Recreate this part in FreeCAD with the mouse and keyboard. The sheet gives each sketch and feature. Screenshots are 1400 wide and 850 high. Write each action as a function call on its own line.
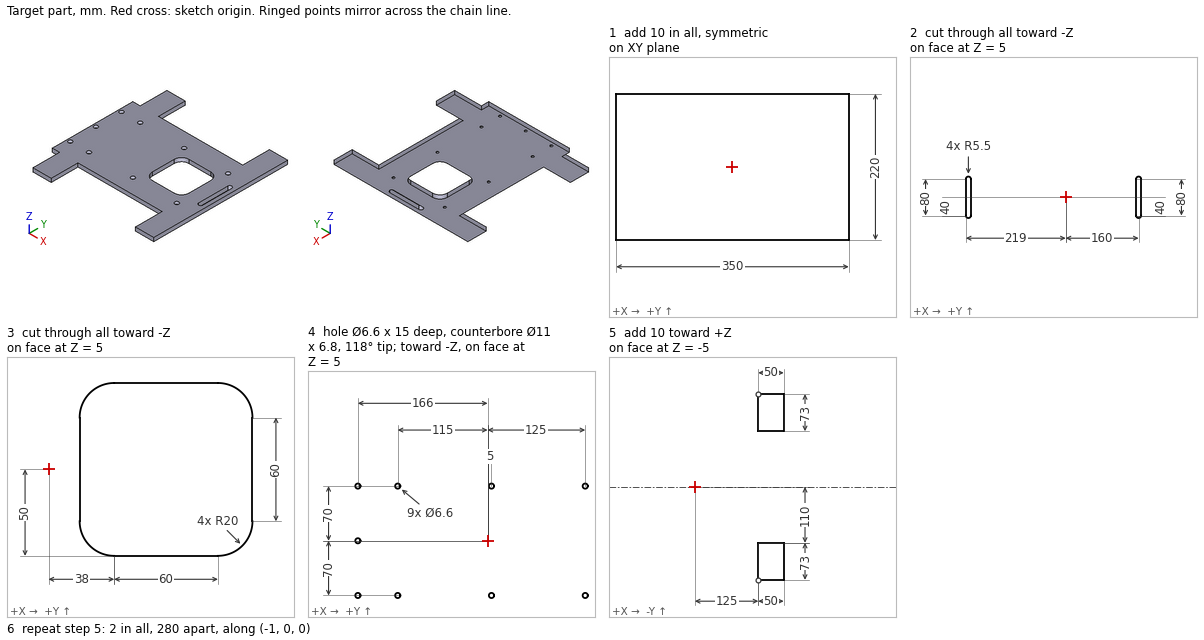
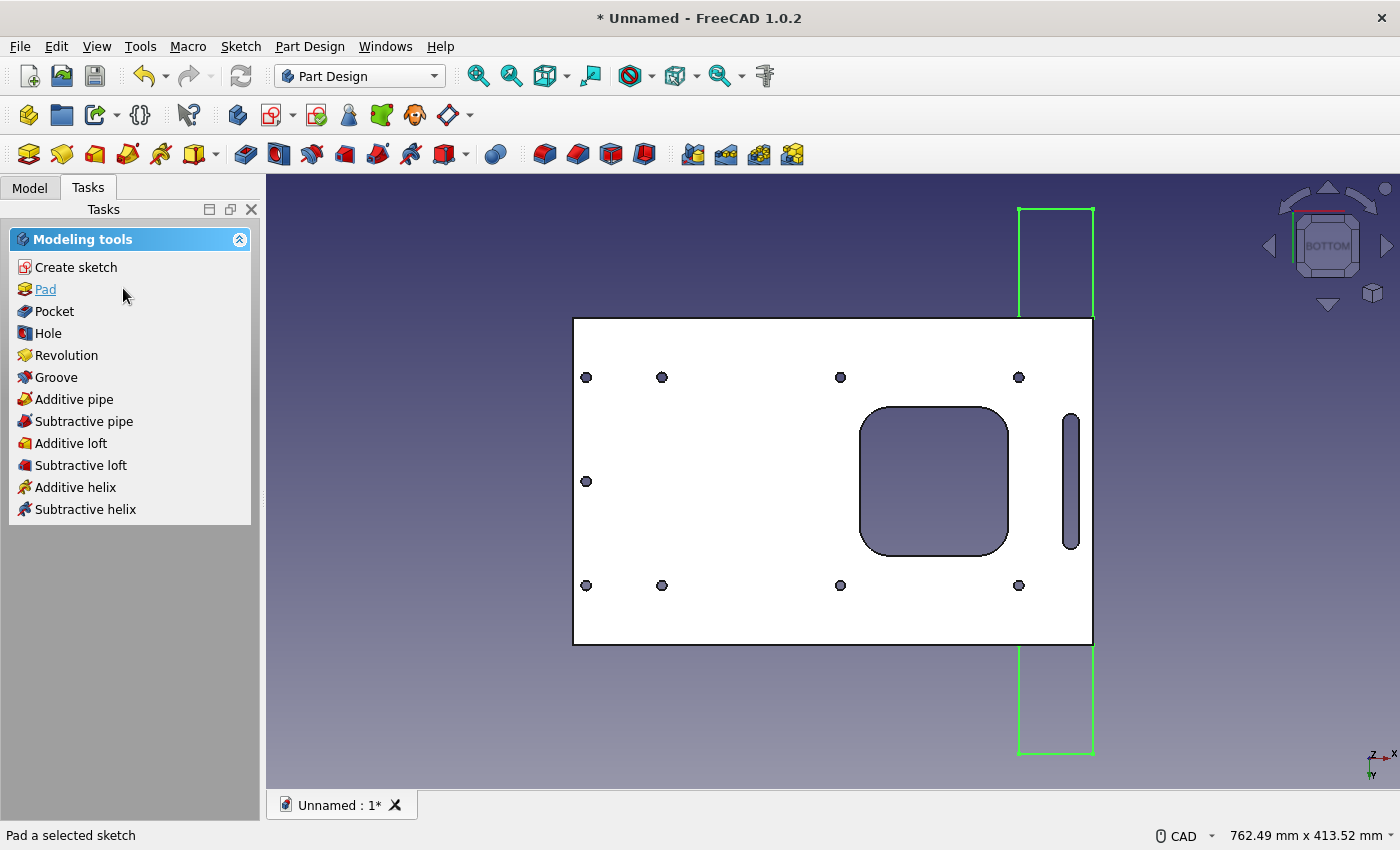
click(29, 154)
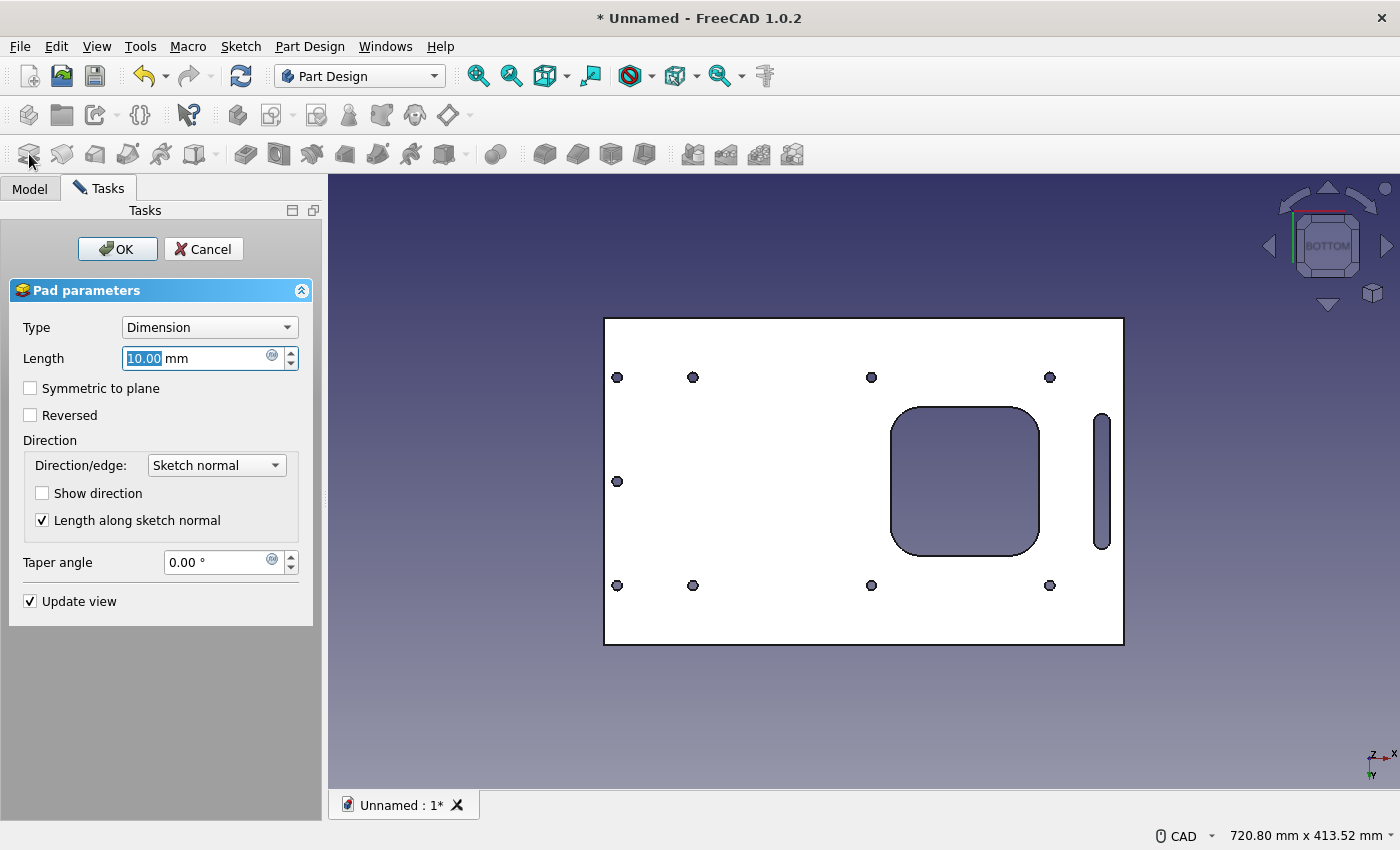
text(10)
key(Tab)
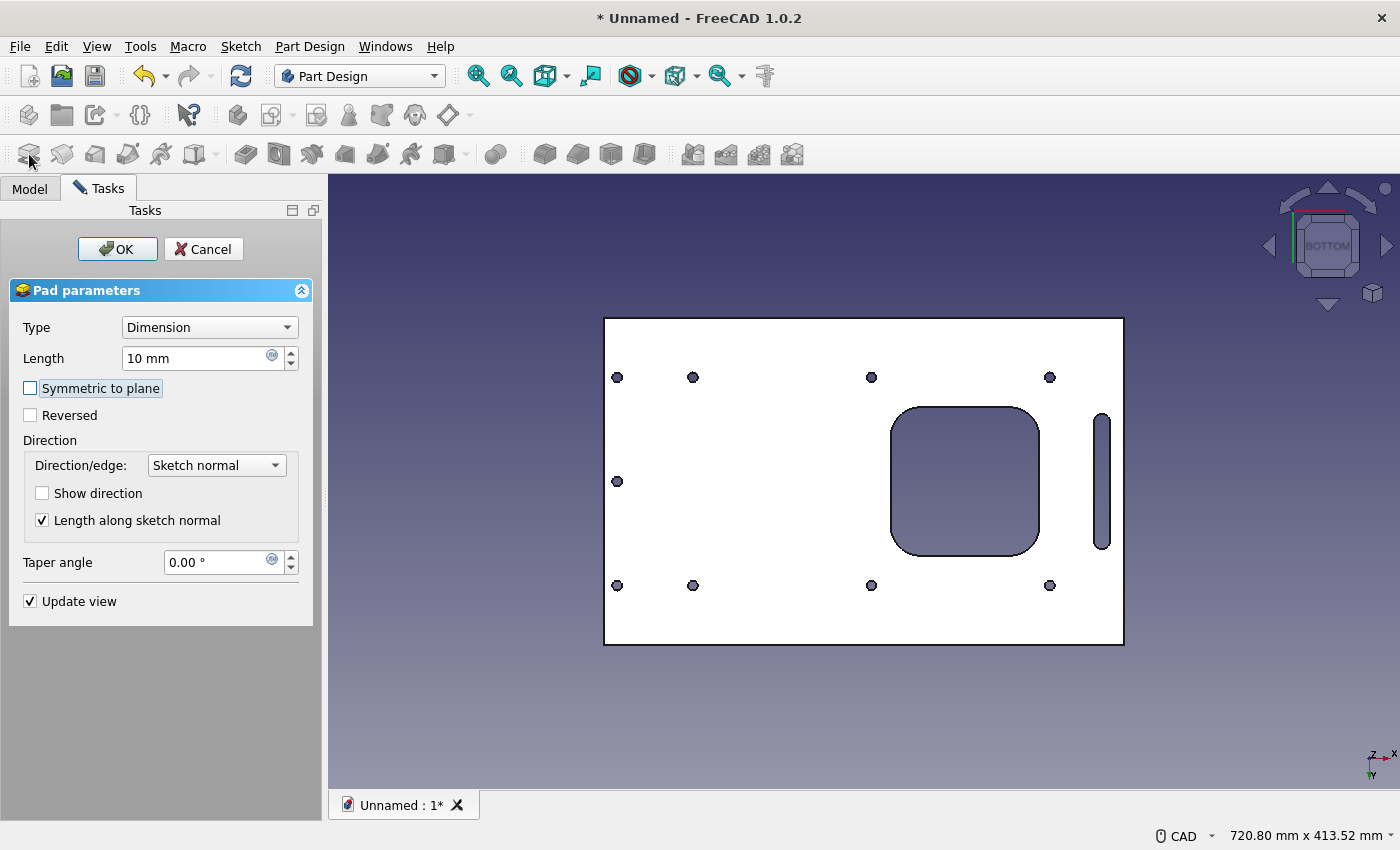
click(31, 415)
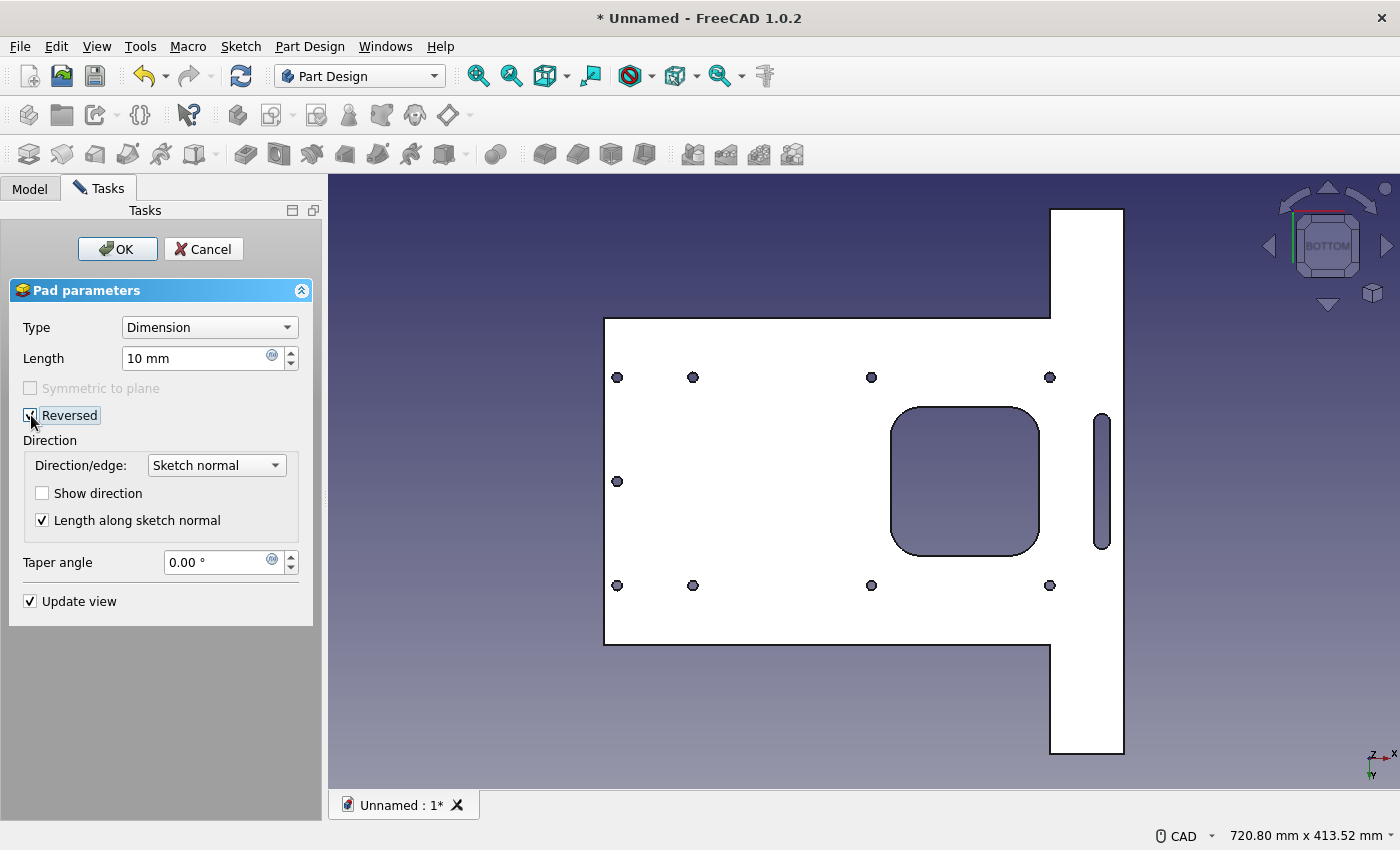
click(118, 249)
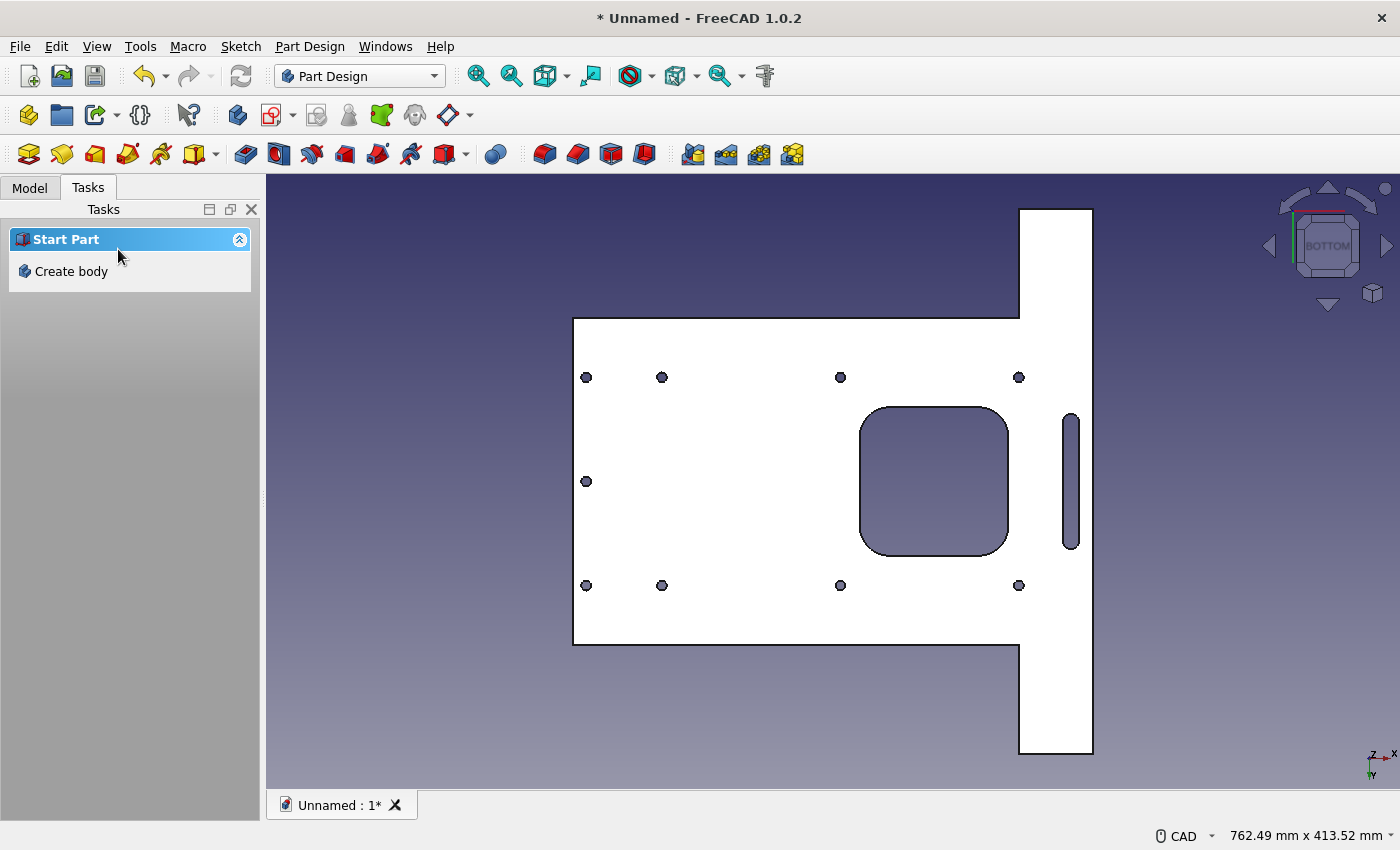
click(30, 188)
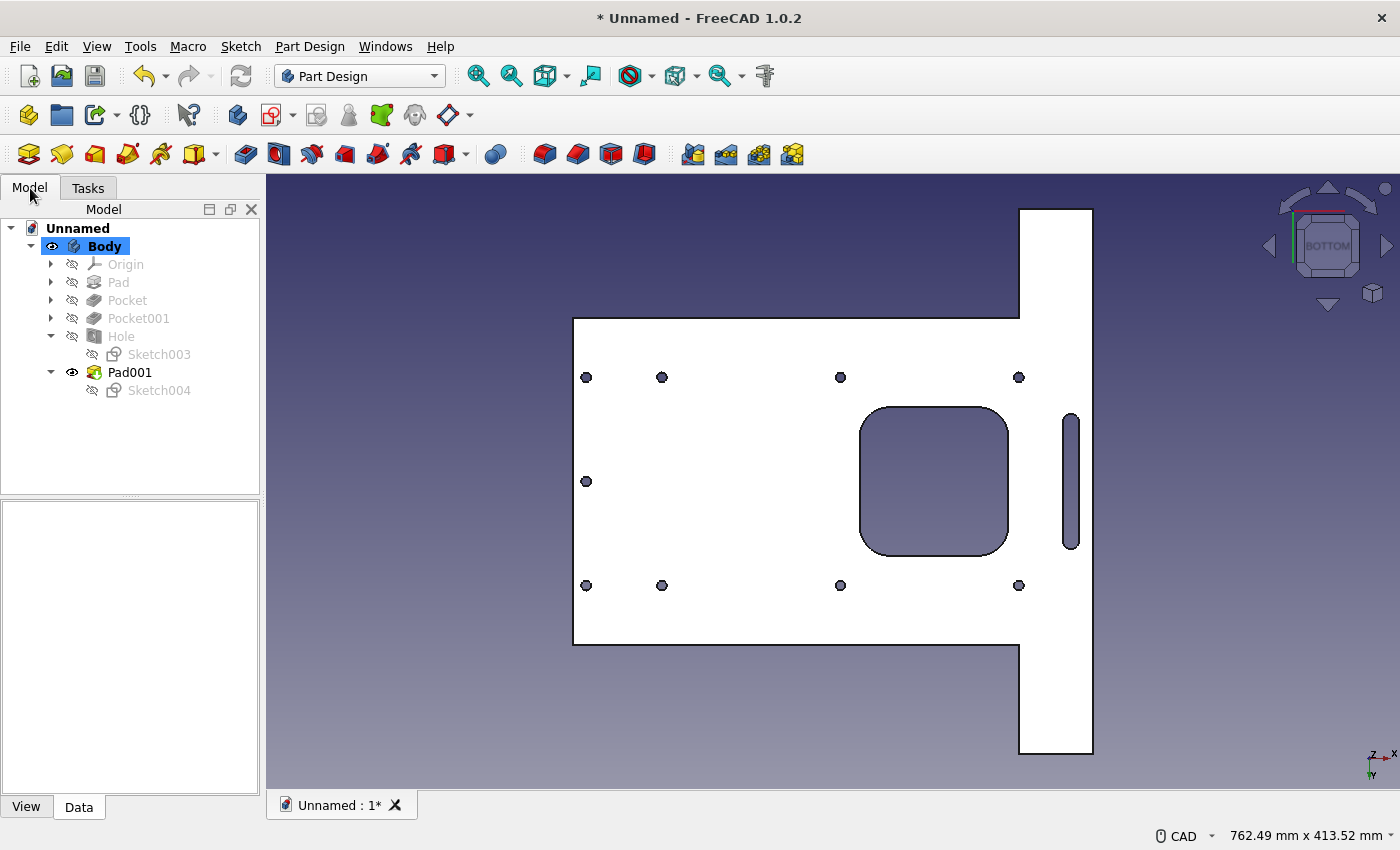
click(117, 372)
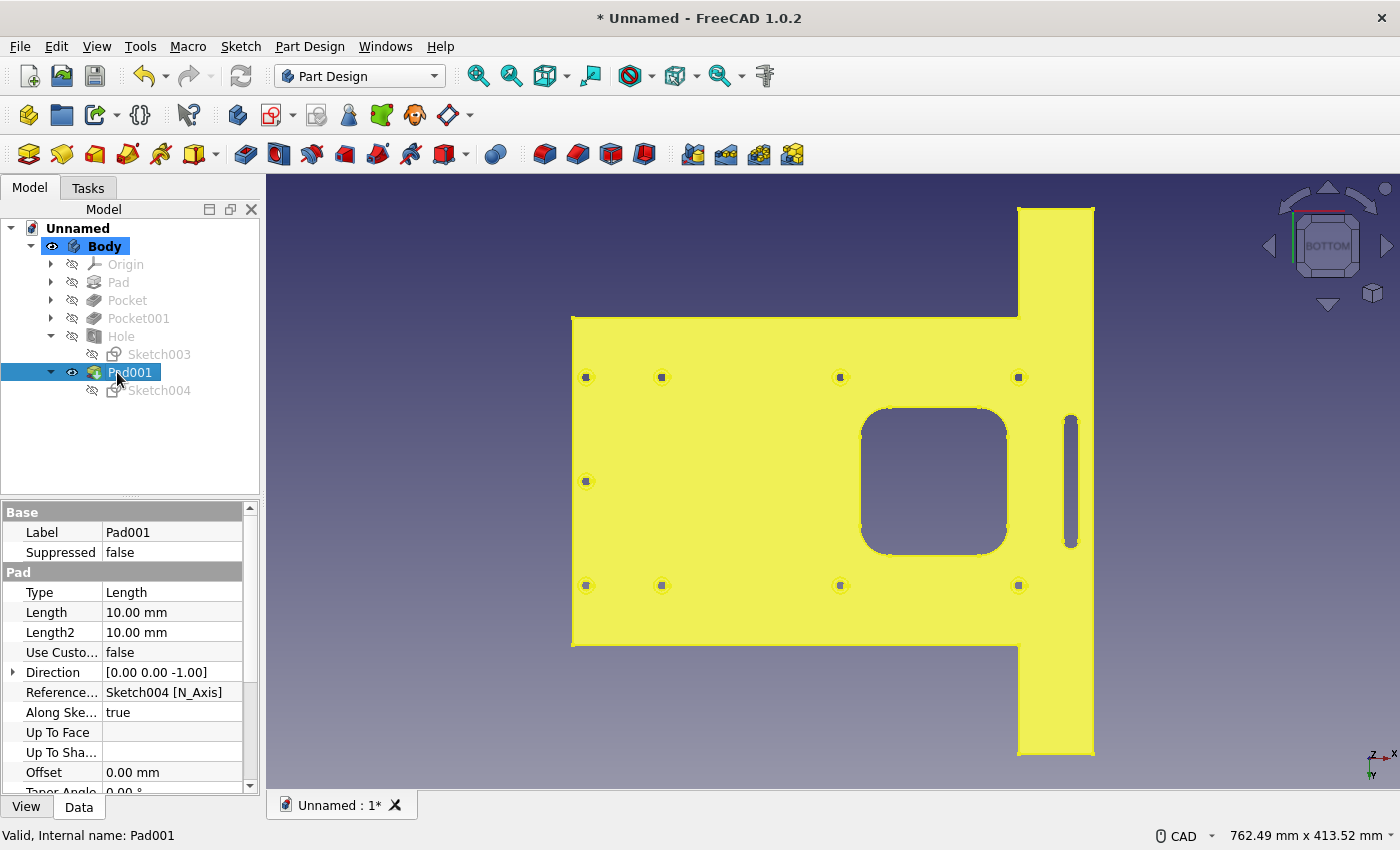
click(726, 154)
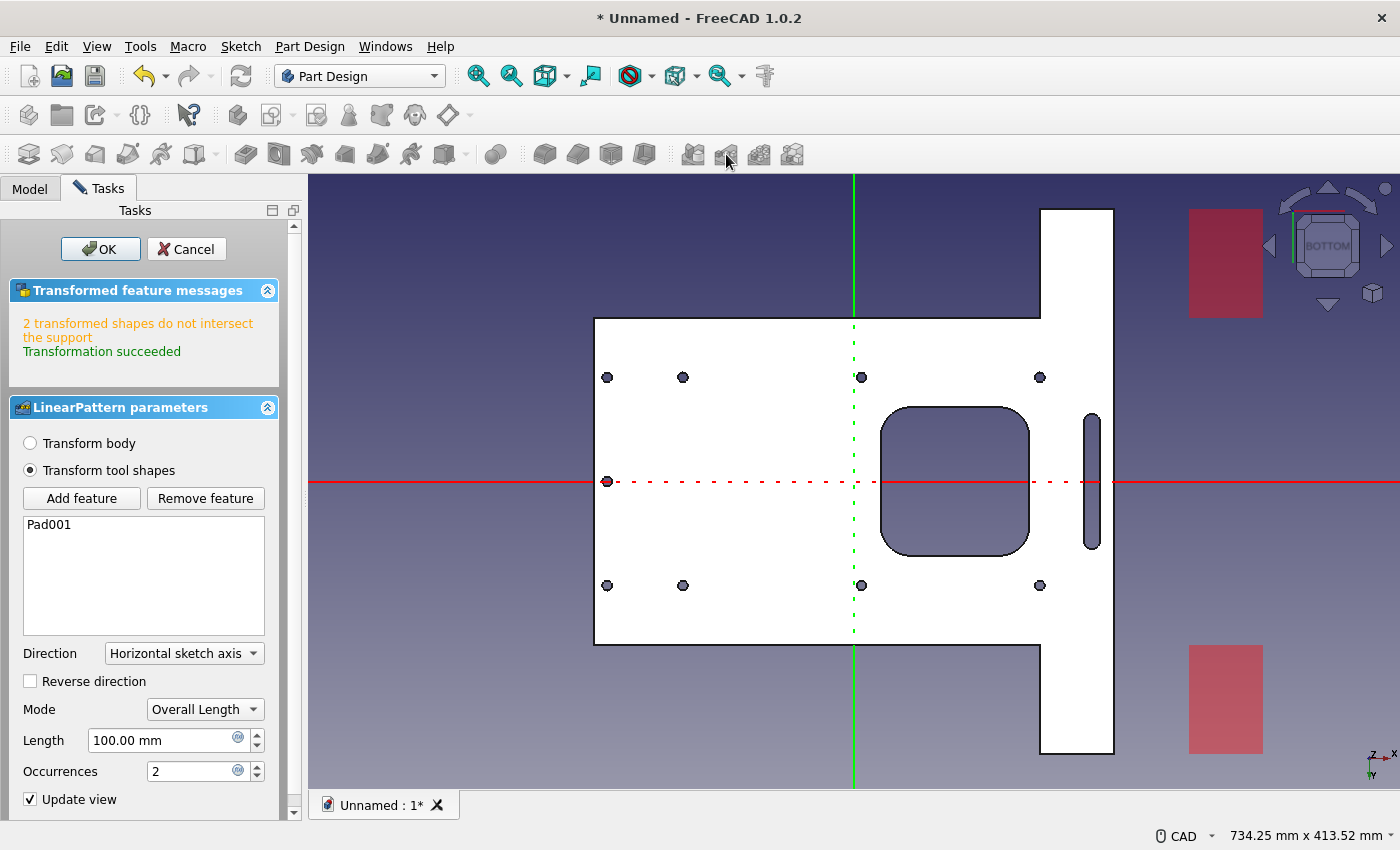
click(185, 654)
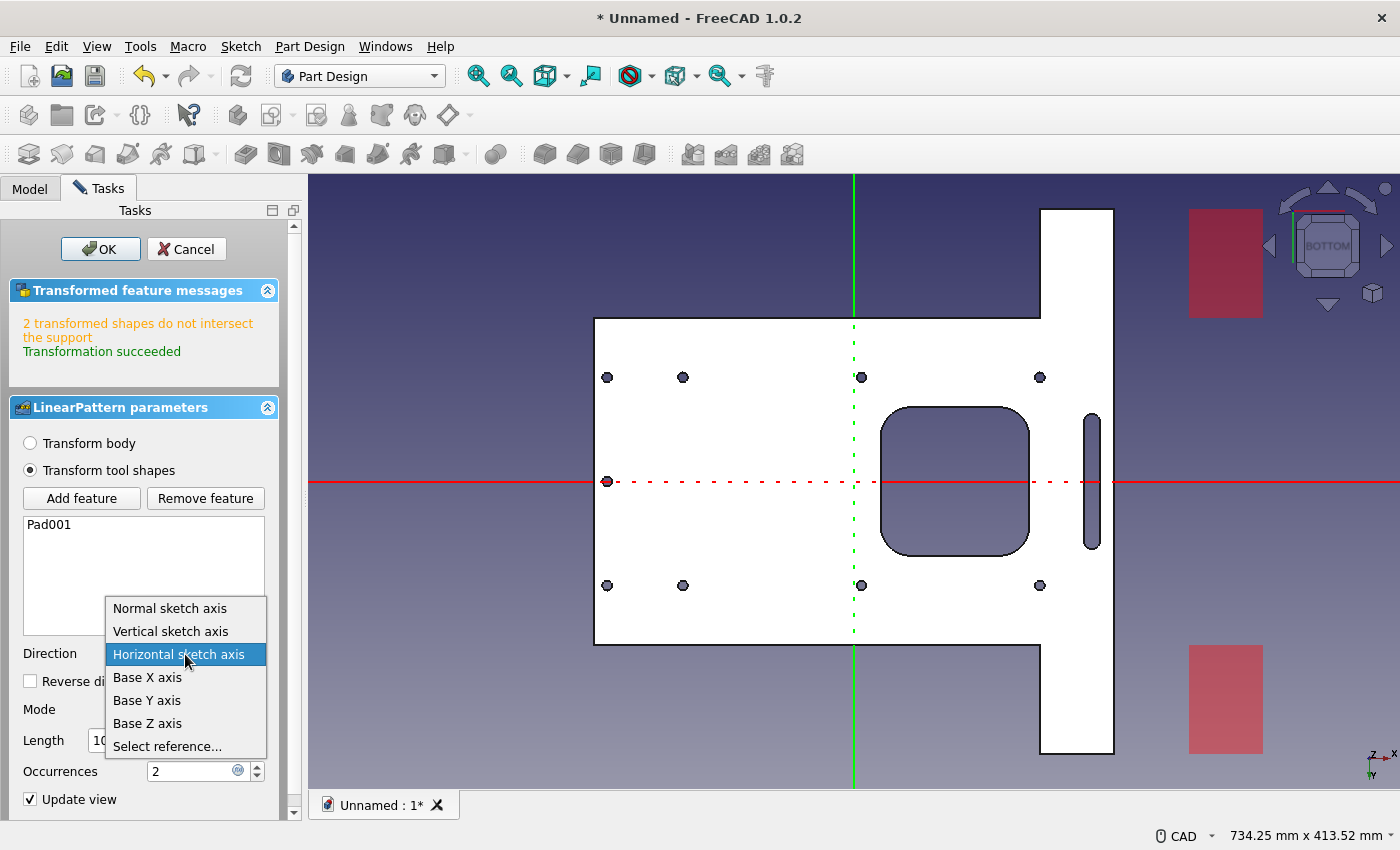
click(184, 678)